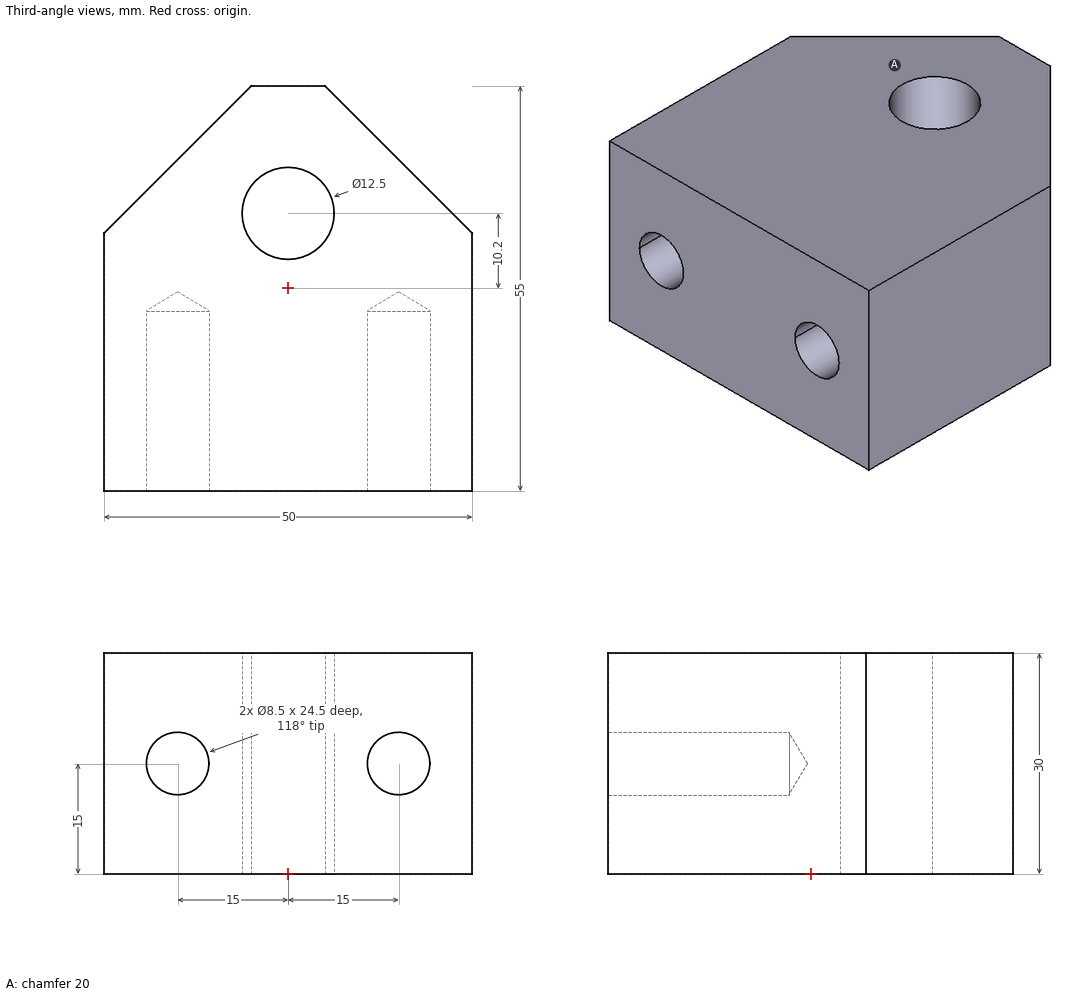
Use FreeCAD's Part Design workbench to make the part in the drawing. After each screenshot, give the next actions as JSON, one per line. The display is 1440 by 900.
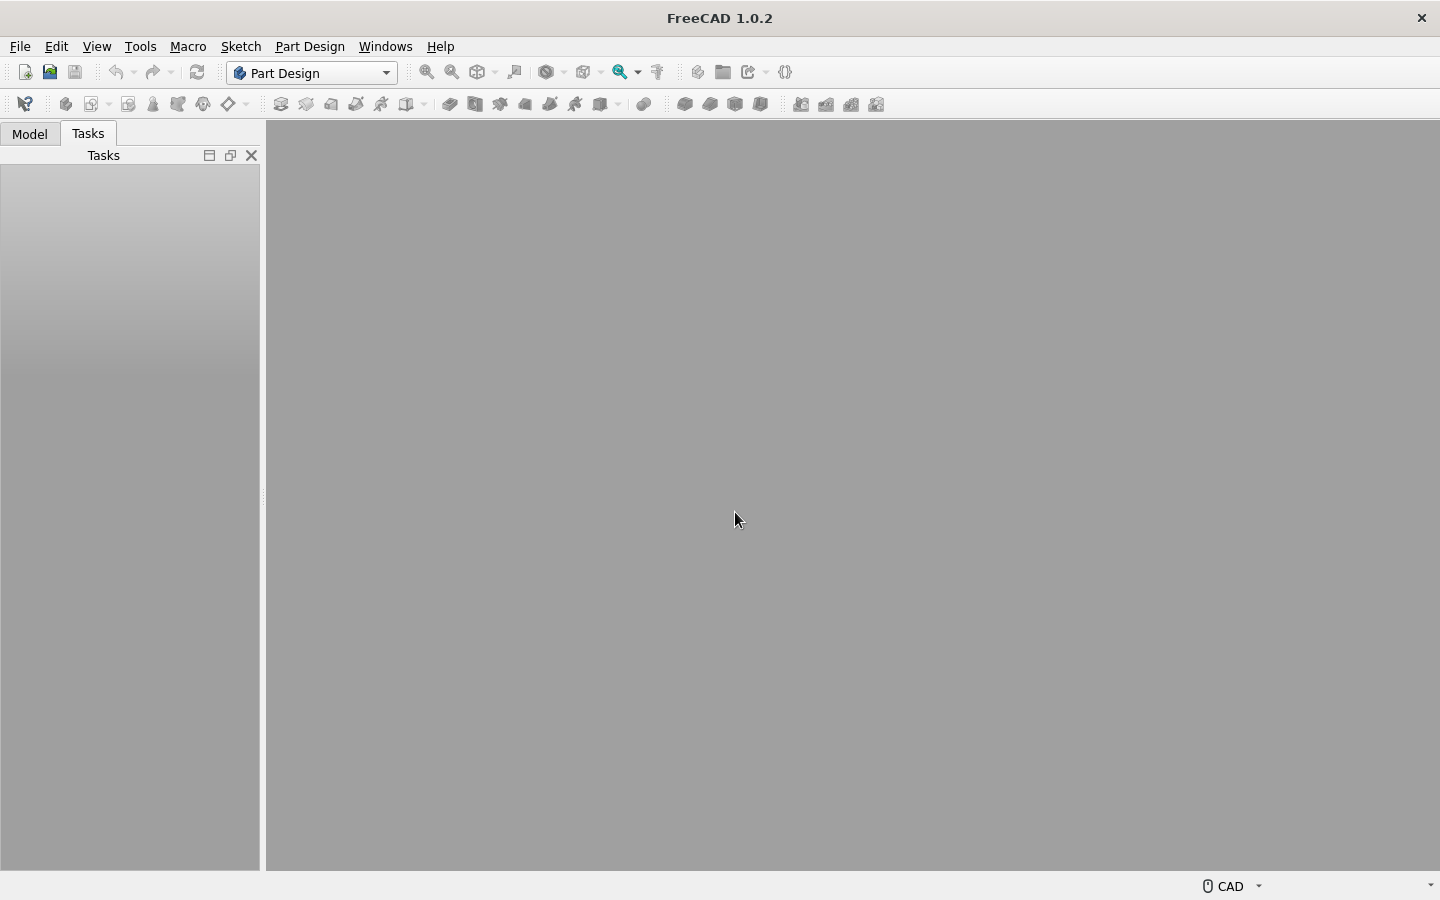
{"action": "key", "text": "ctrl+n"}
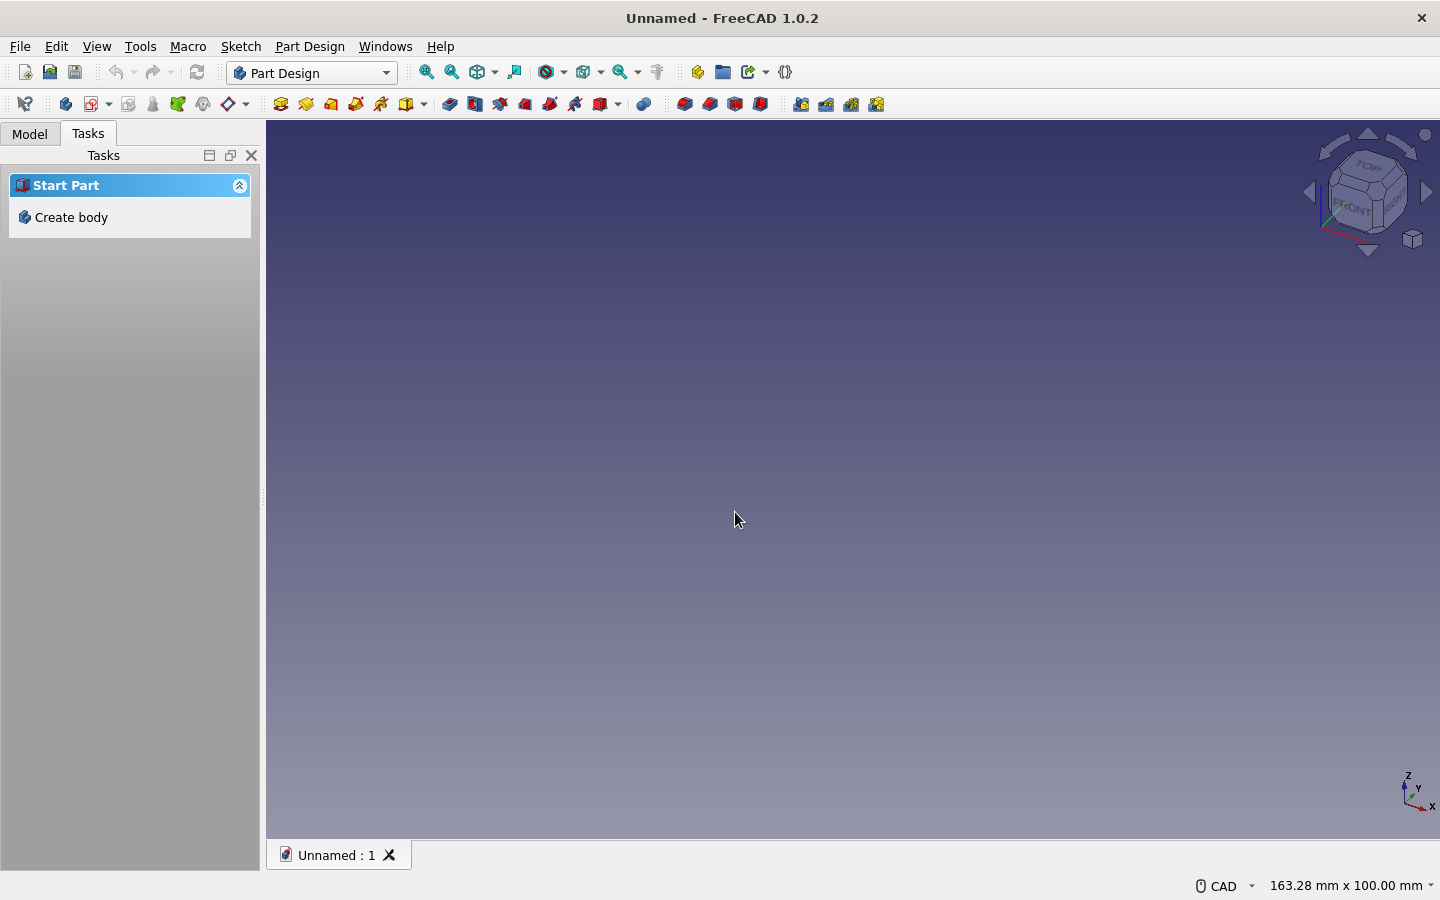
{"action": "left_click", "coordinate": [90, 104]}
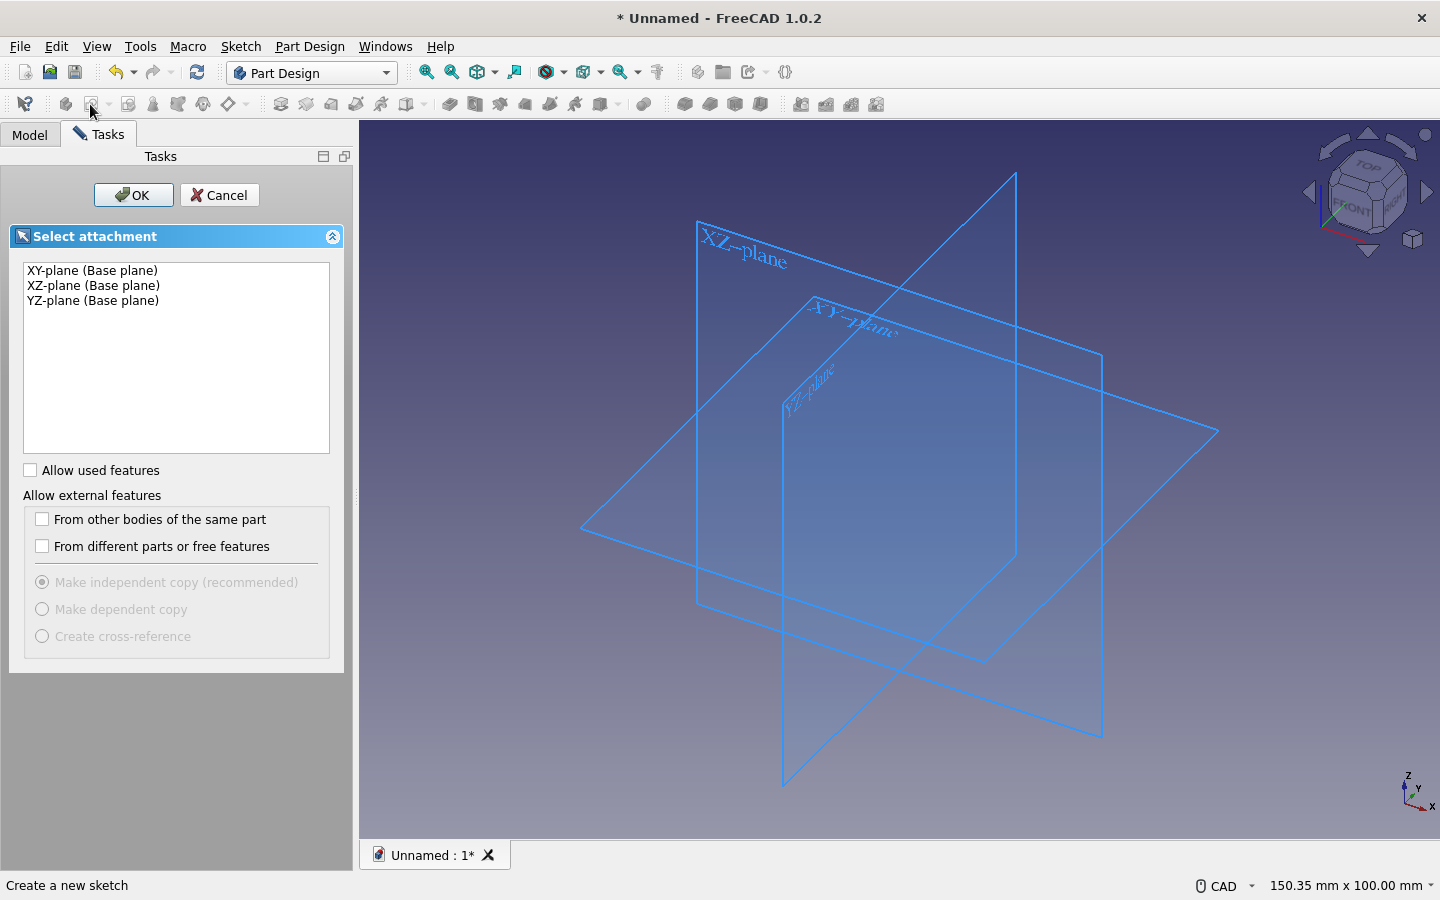
{"action": "left_click", "coordinate": [84, 270]}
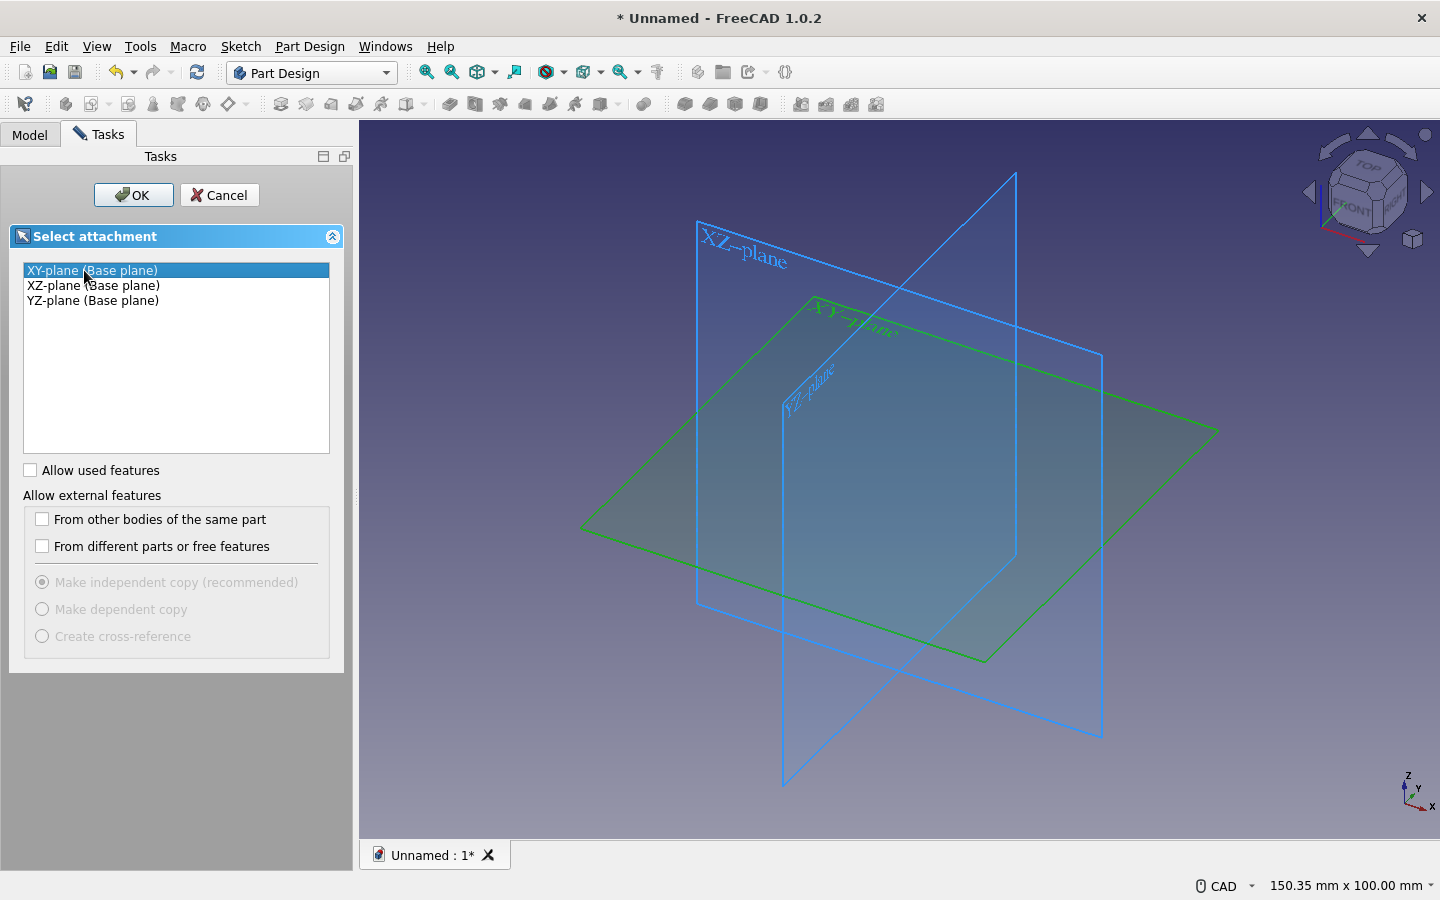
{"action": "left_click", "coordinate": [134, 195]}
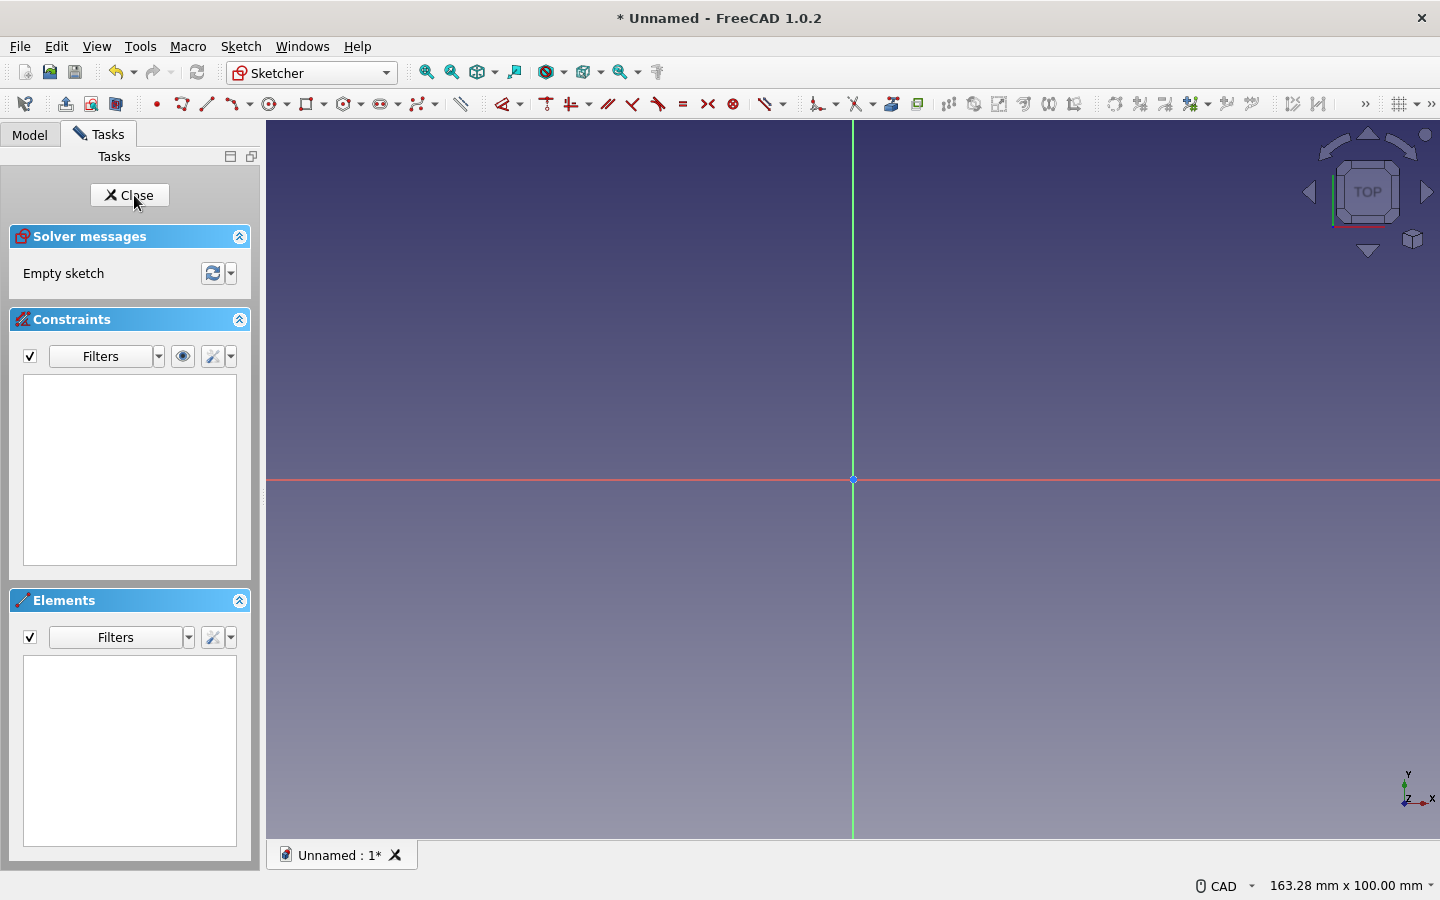
{"action": "left_click", "coordinate": [324, 104]}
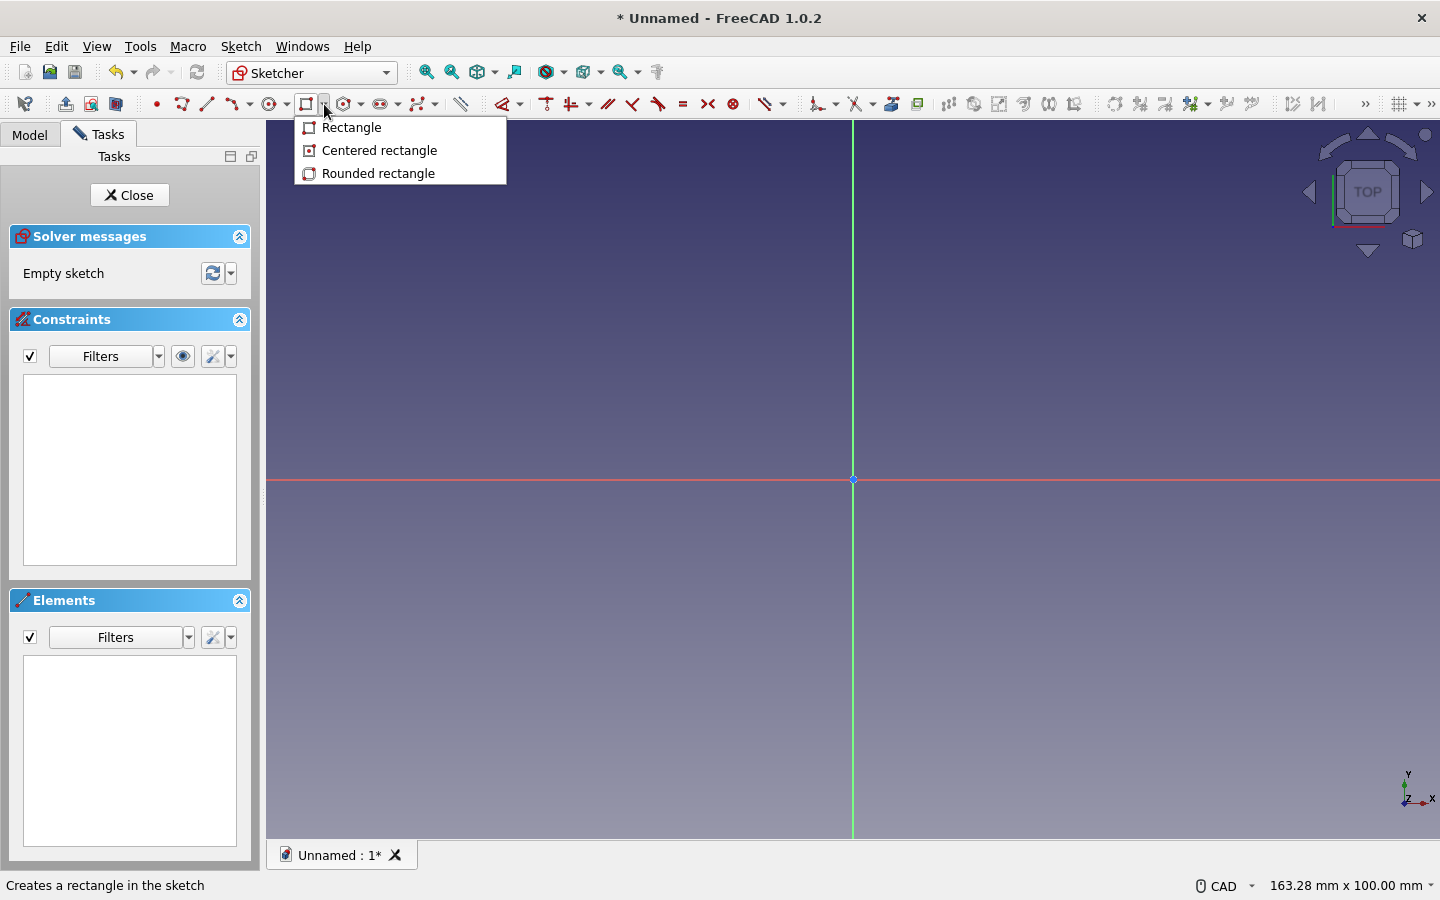
{"action": "left_click", "coordinate": [400, 150]}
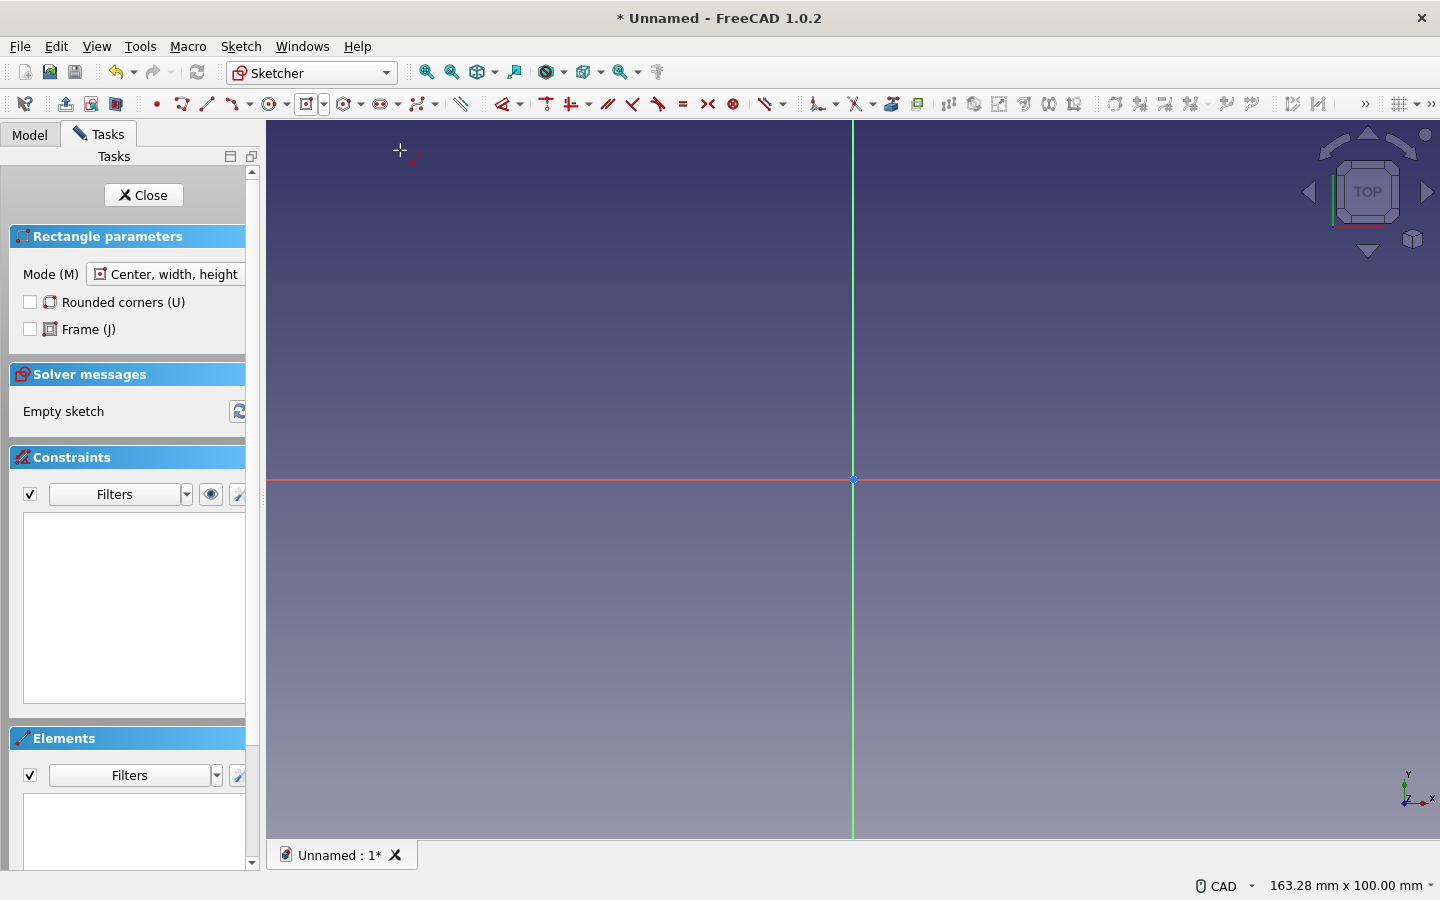
{"action": "left_click", "coordinate": [853, 480]}
{"action": "mouse_move", "coordinate": [1033, 282]}